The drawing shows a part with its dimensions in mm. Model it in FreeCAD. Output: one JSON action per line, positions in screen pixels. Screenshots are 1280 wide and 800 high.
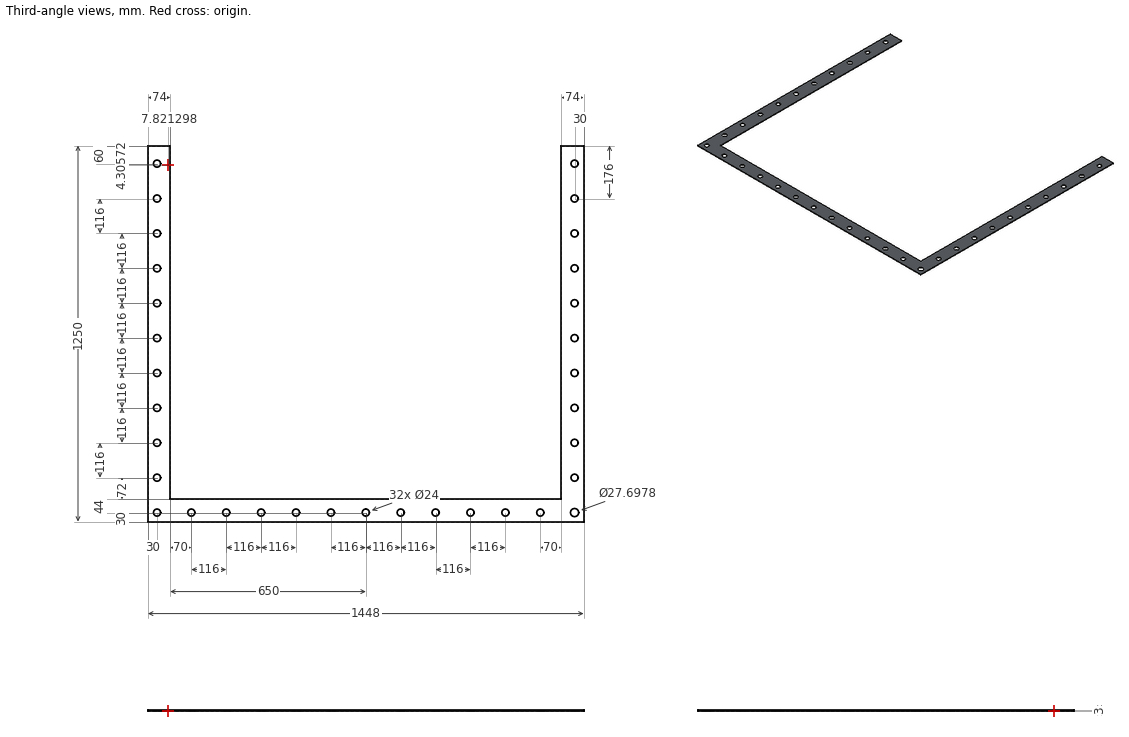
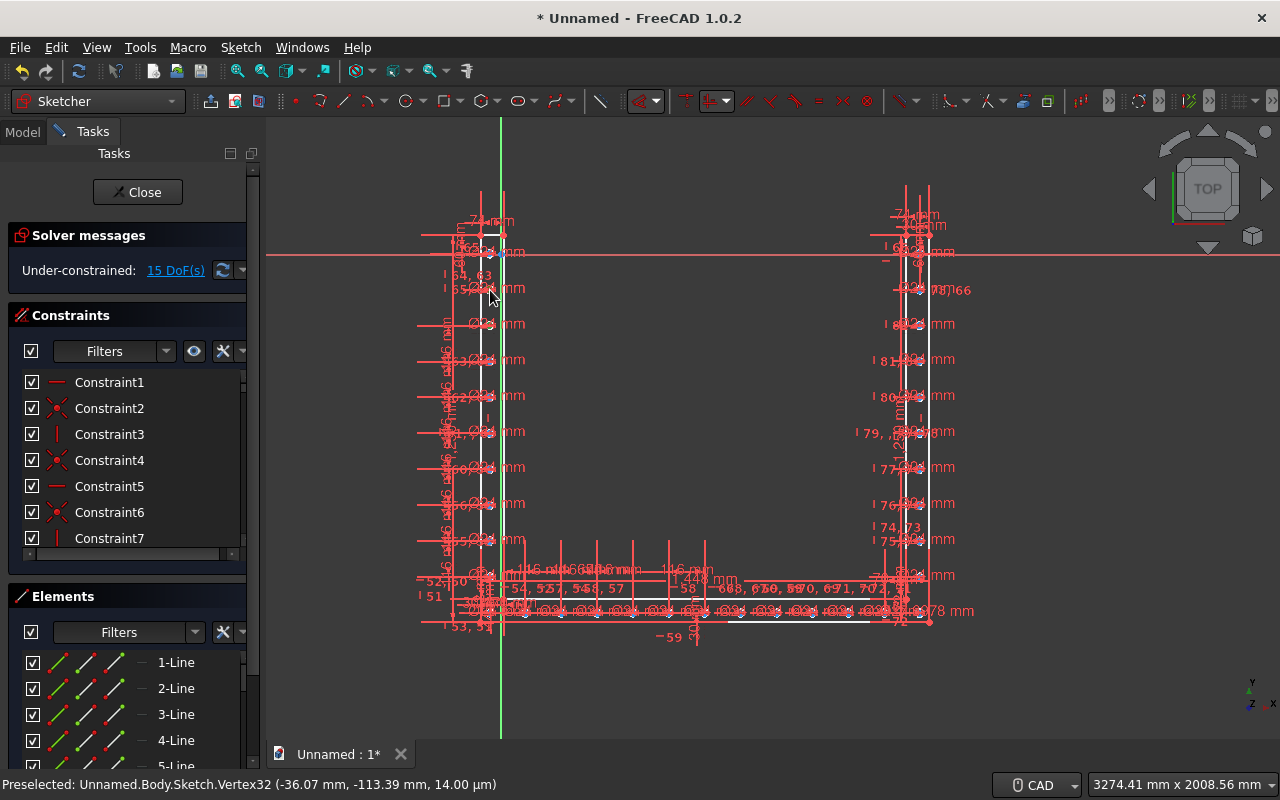
{"action": "key", "text": "i"}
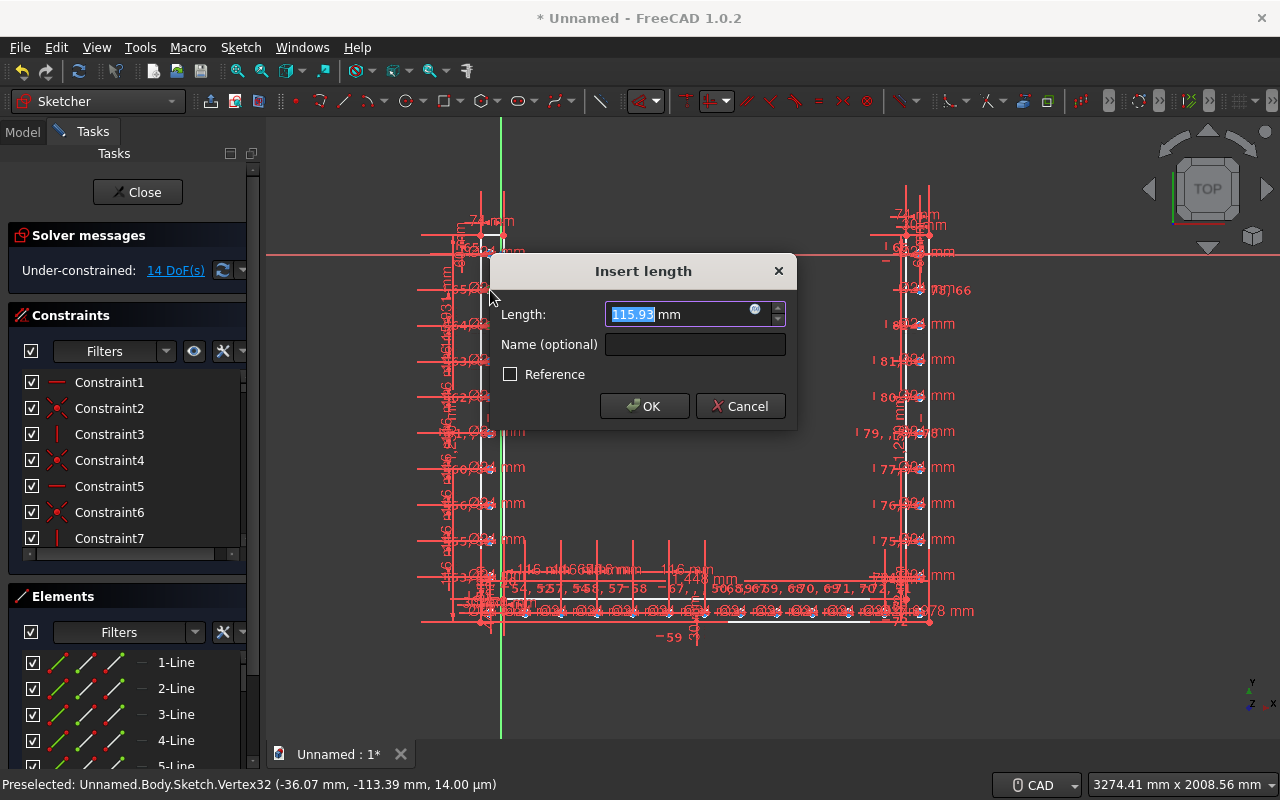
{"action": "type", "text": "116"}
{"action": "key", "text": "Return"}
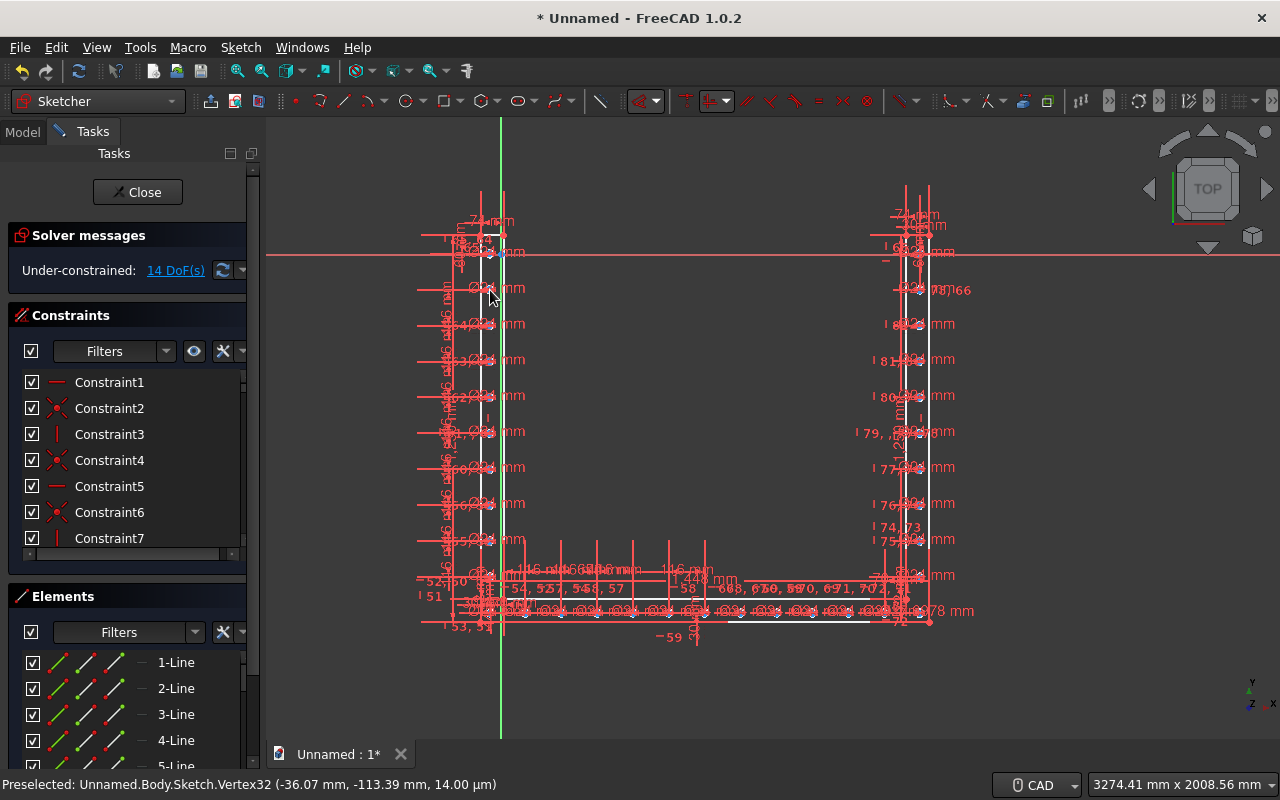
{"action": "left_click", "coordinate": [929, 235]}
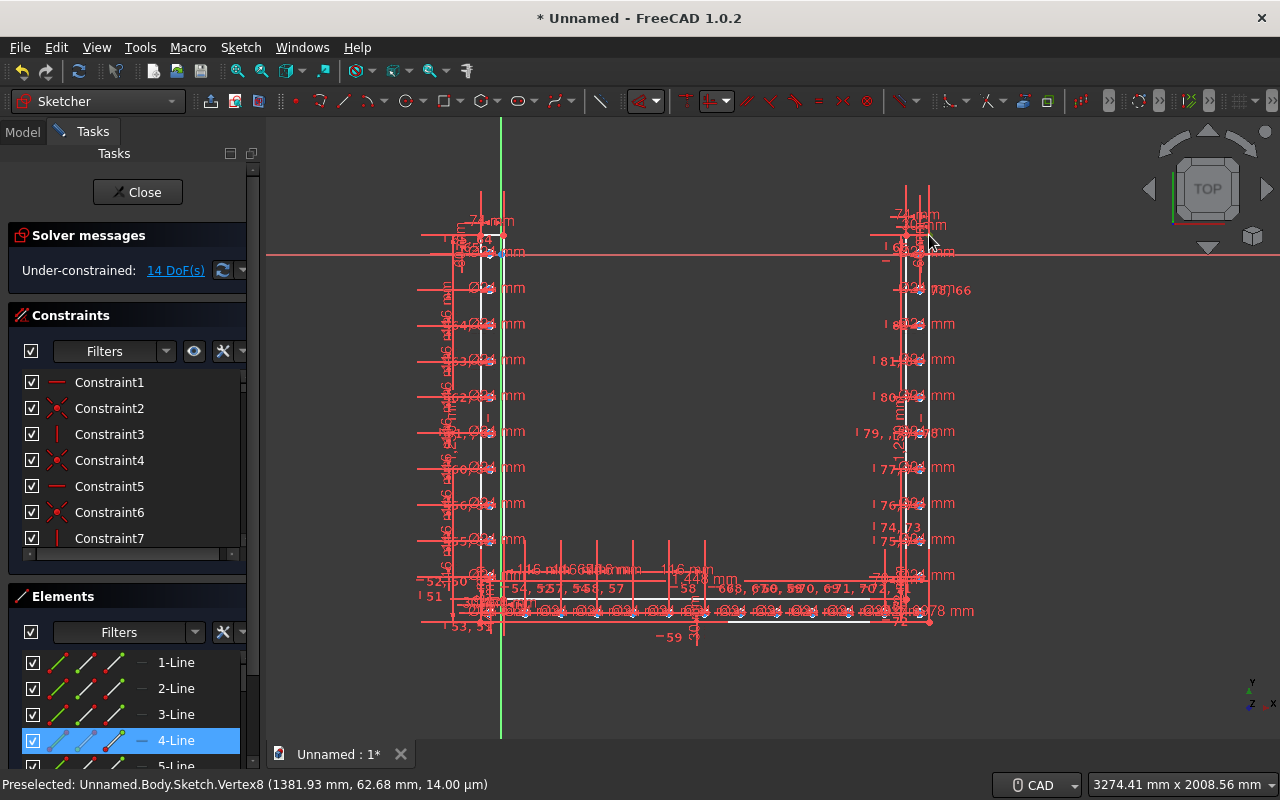
{"action": "left_click", "coordinate": [920, 290]}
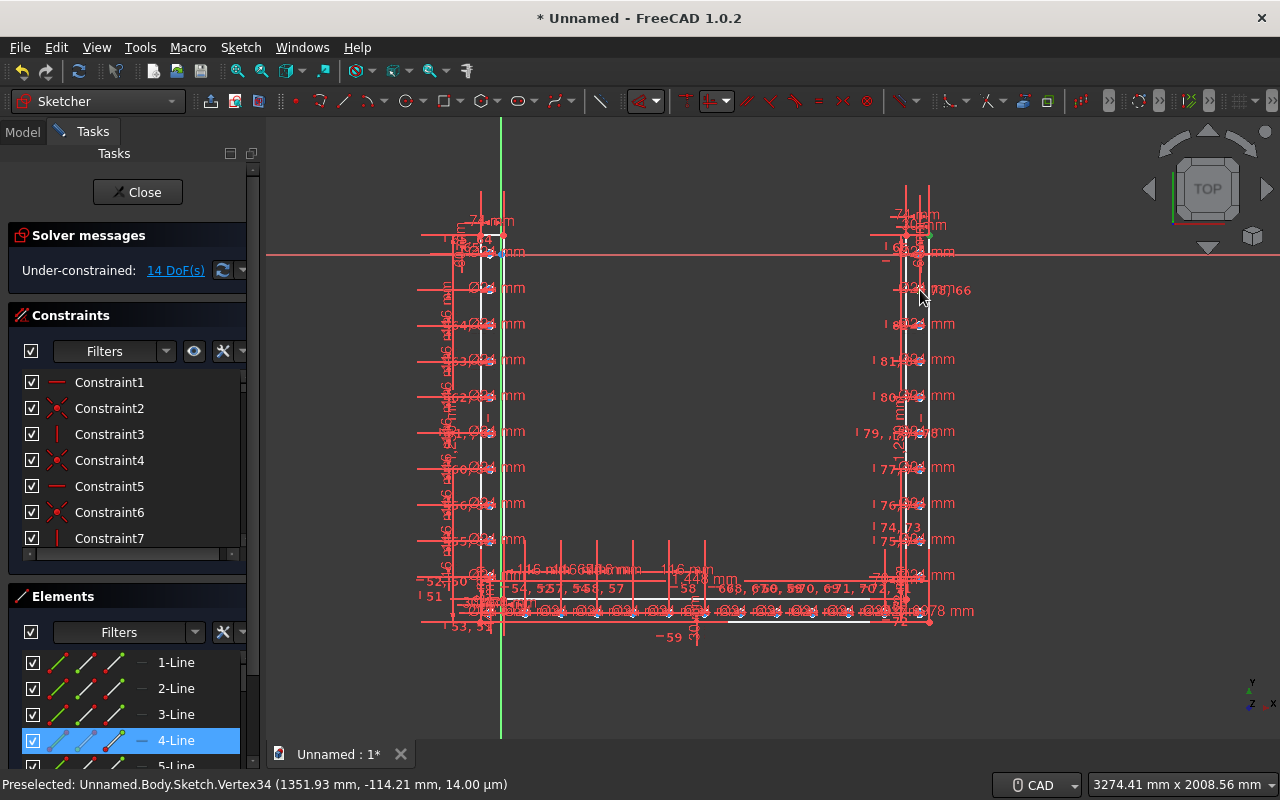
{"action": "left_click", "coordinate": [658, 102]}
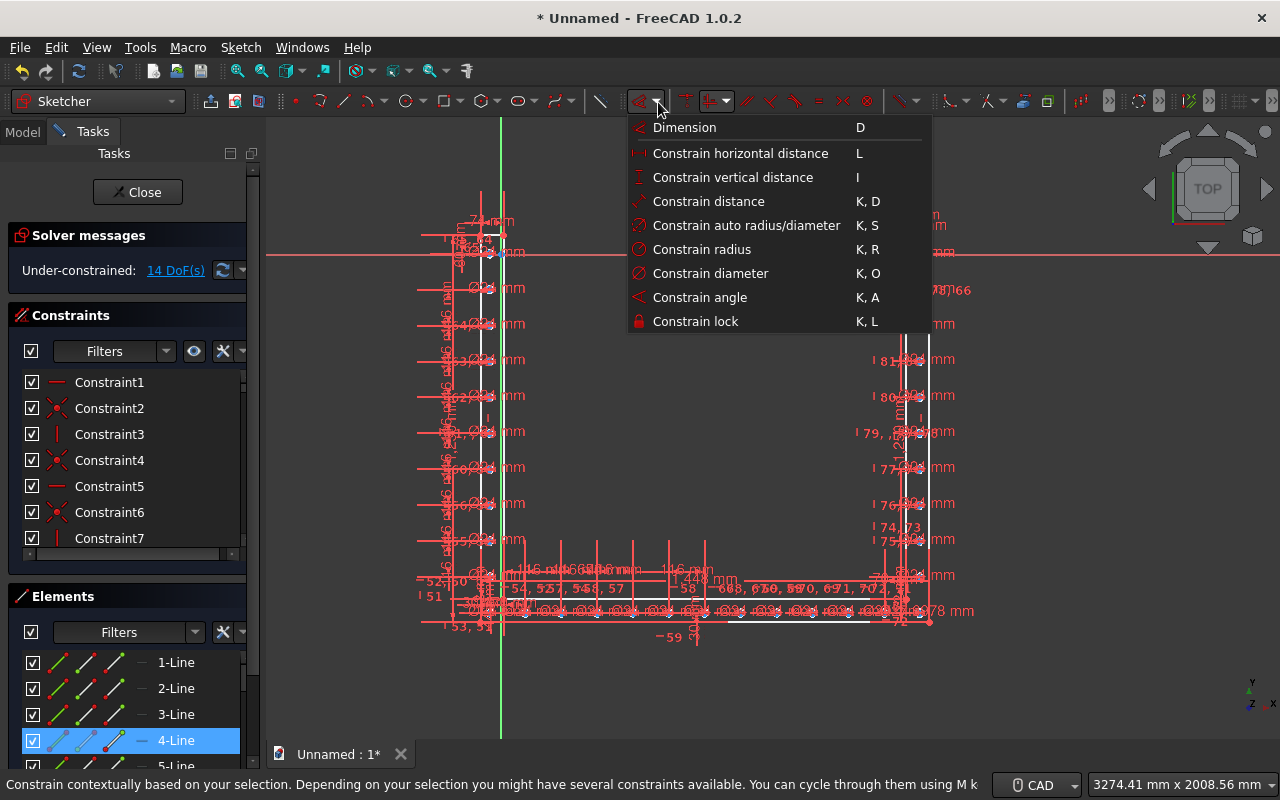
{"action": "left_click", "coordinate": [780, 177]}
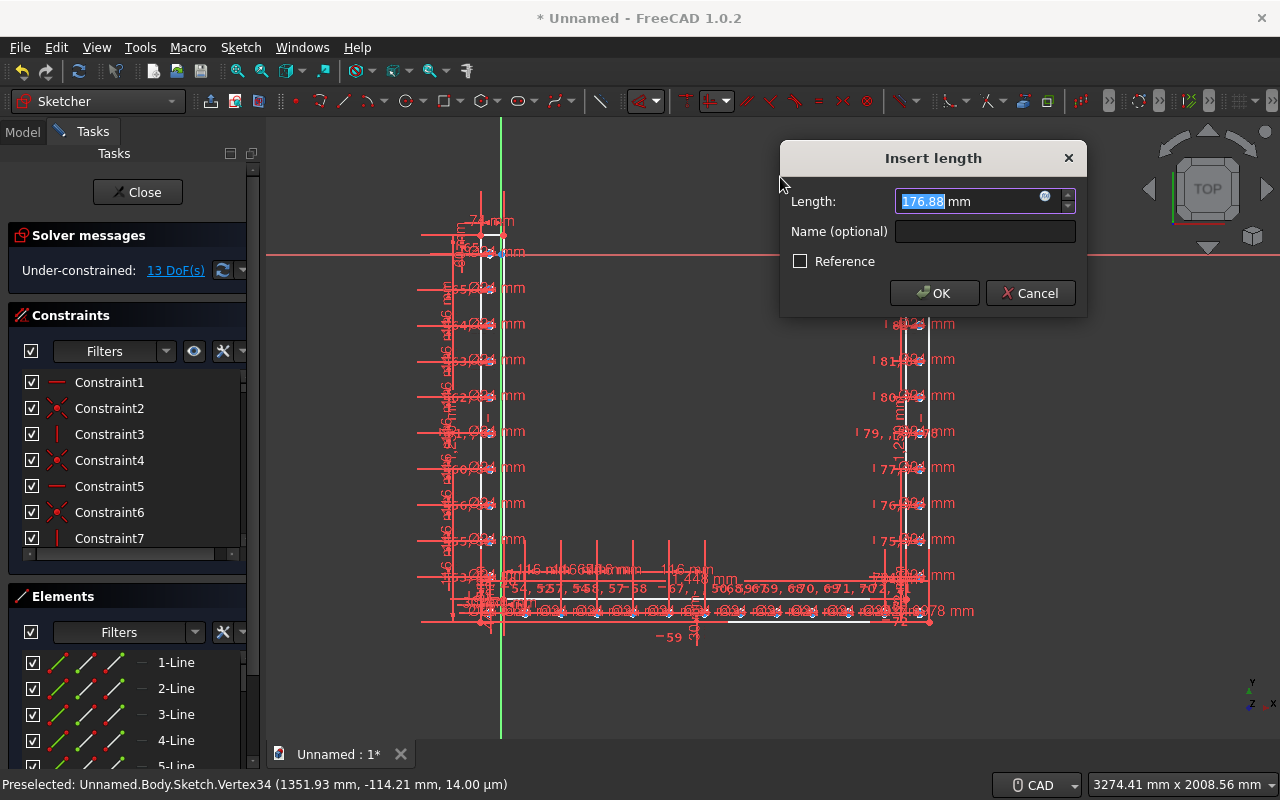
{"action": "type", "text": "176"}
{"action": "key", "text": "Return"}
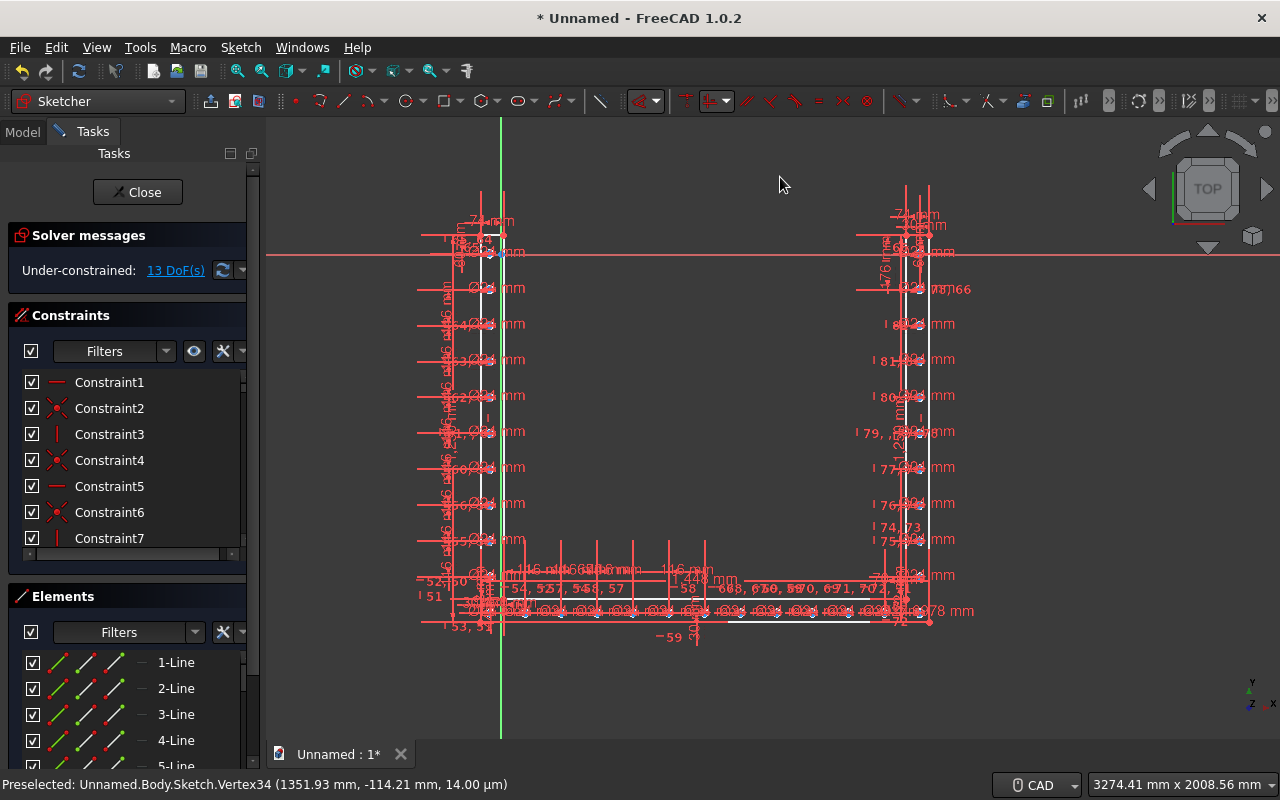
{"action": "left_click", "coordinate": [705, 613]}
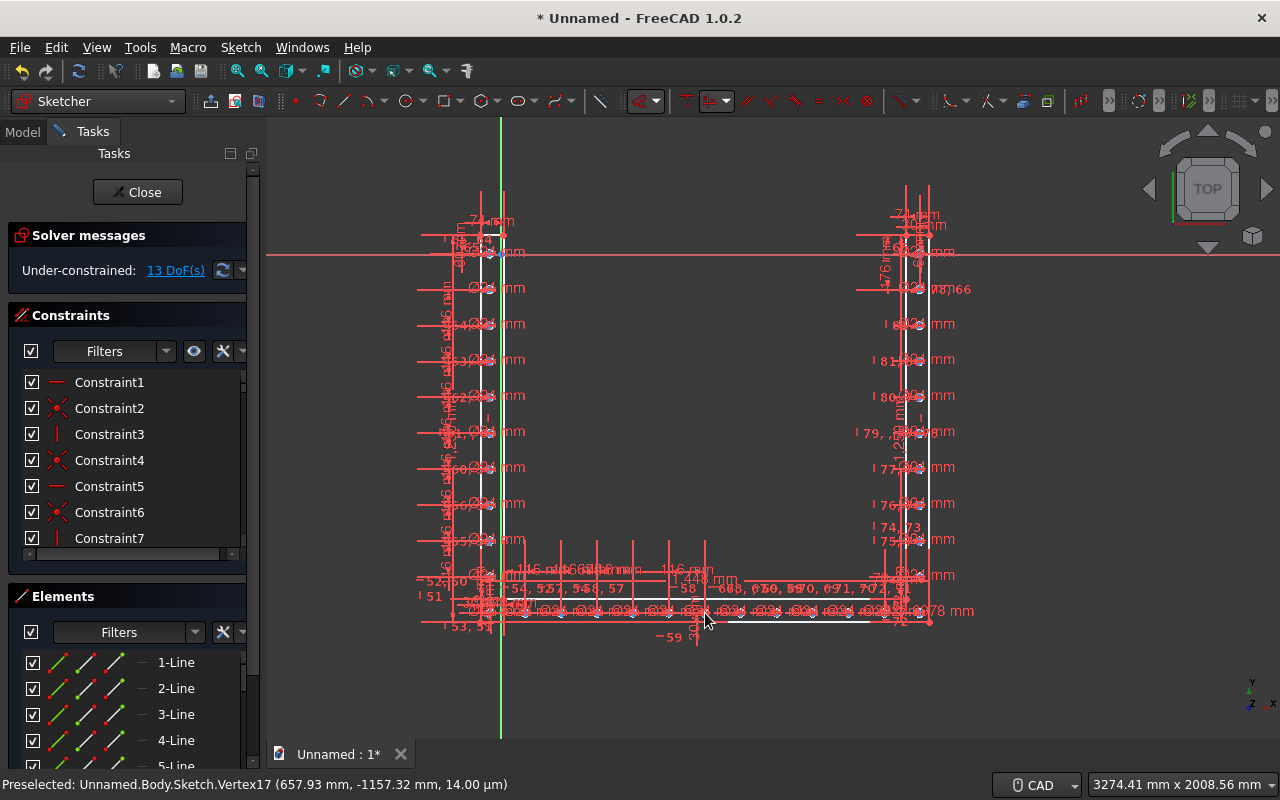
{"action": "left_click", "coordinate": [741, 613]}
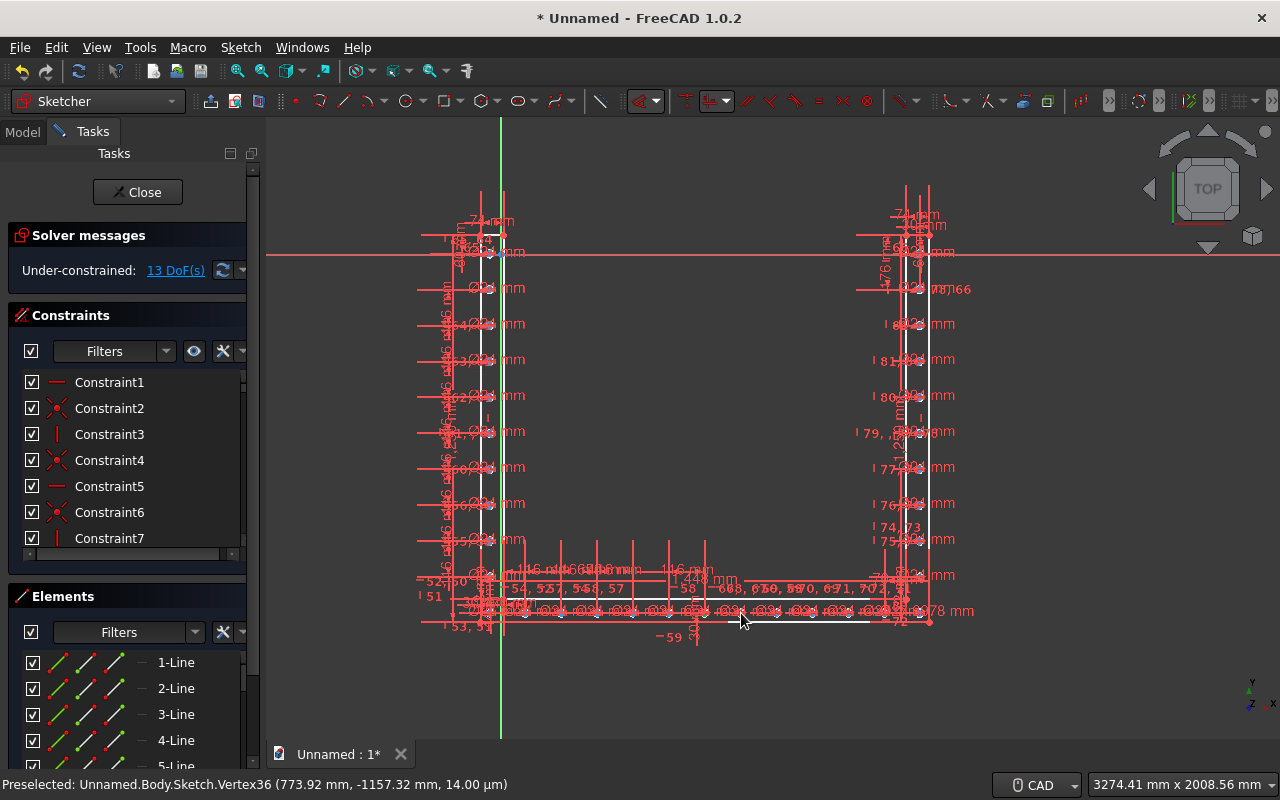
{"action": "key", "text": "l"}